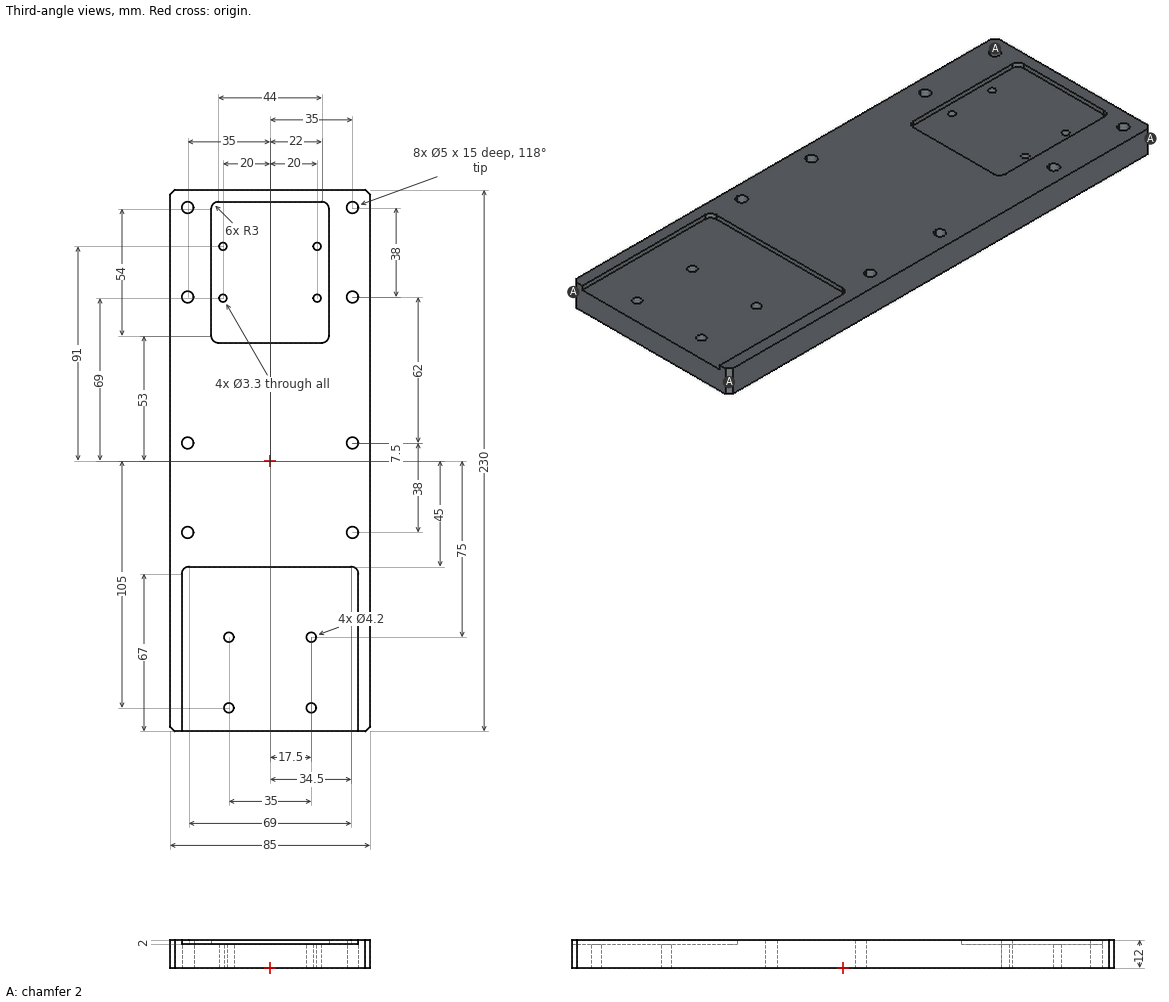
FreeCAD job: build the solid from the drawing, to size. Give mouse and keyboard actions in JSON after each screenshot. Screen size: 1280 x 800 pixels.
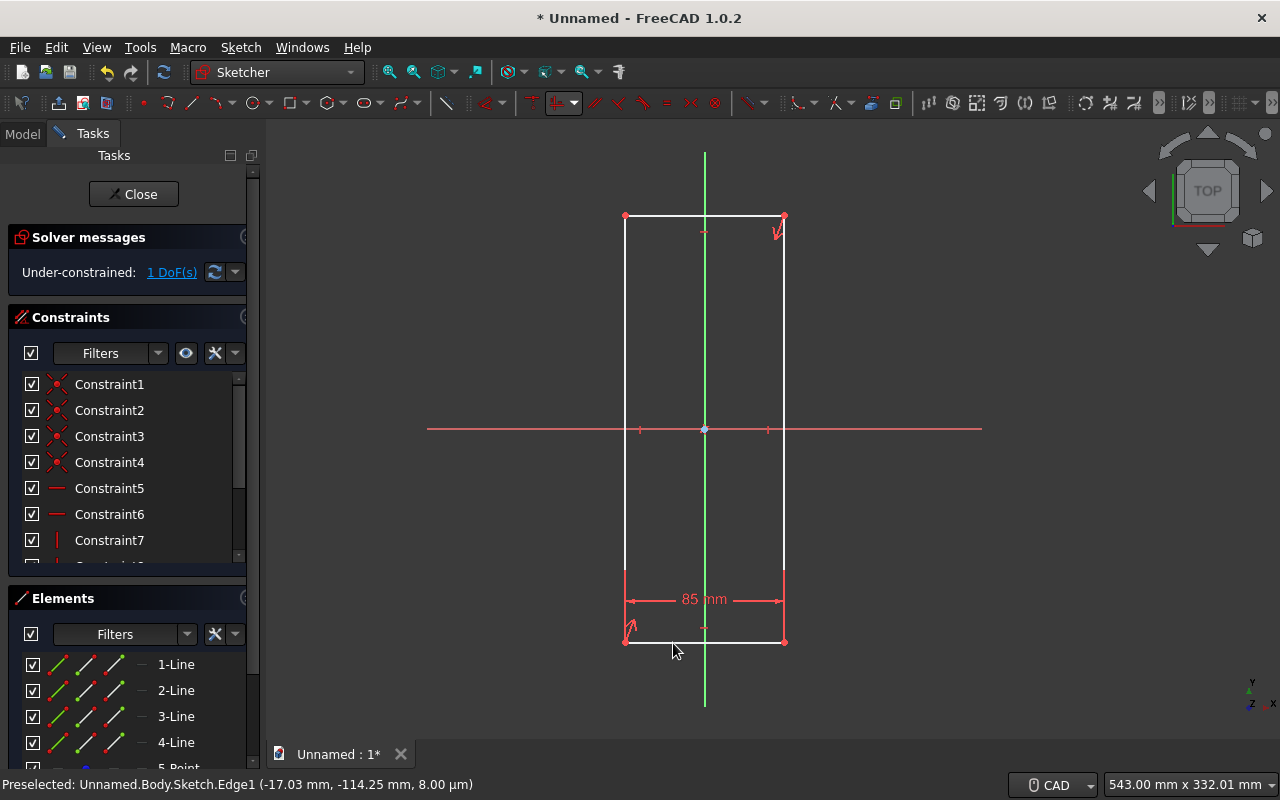
{"action": "left_click", "coordinate": [784, 515]}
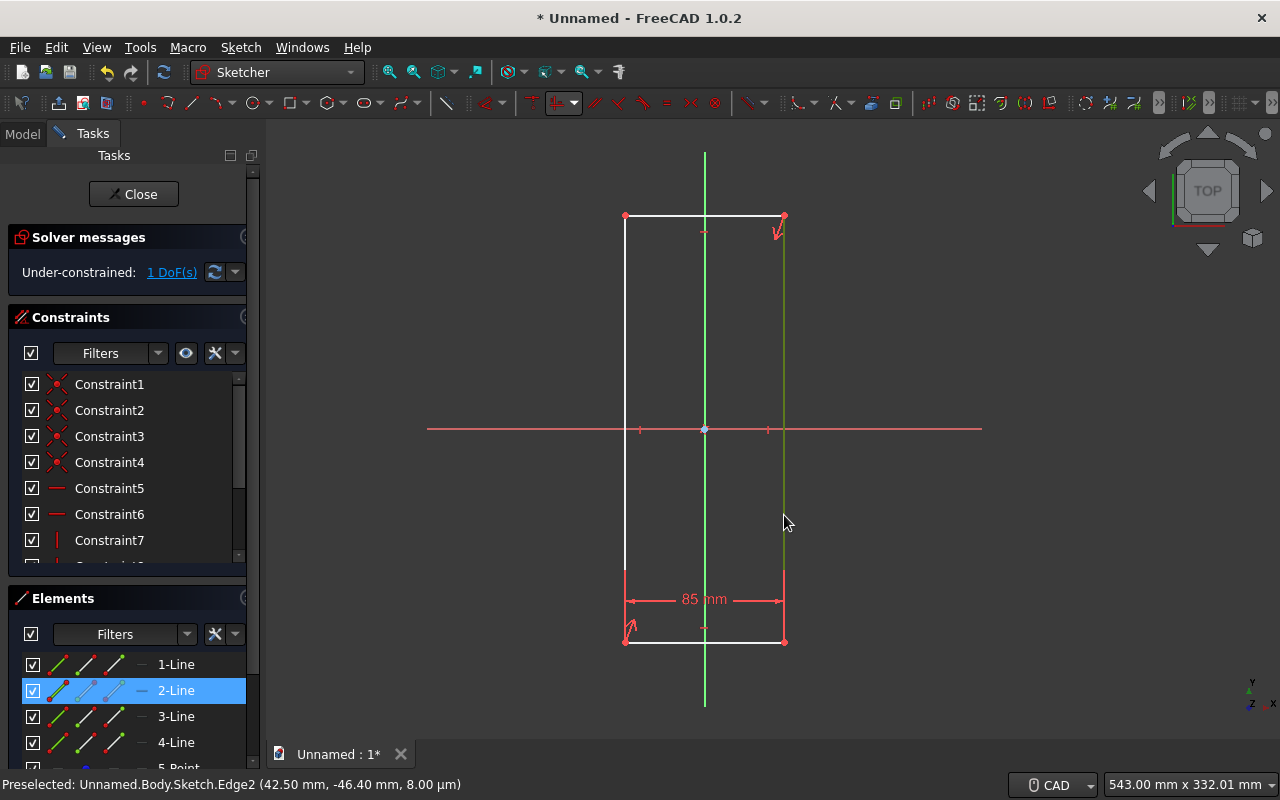
{"action": "key", "text": "i"}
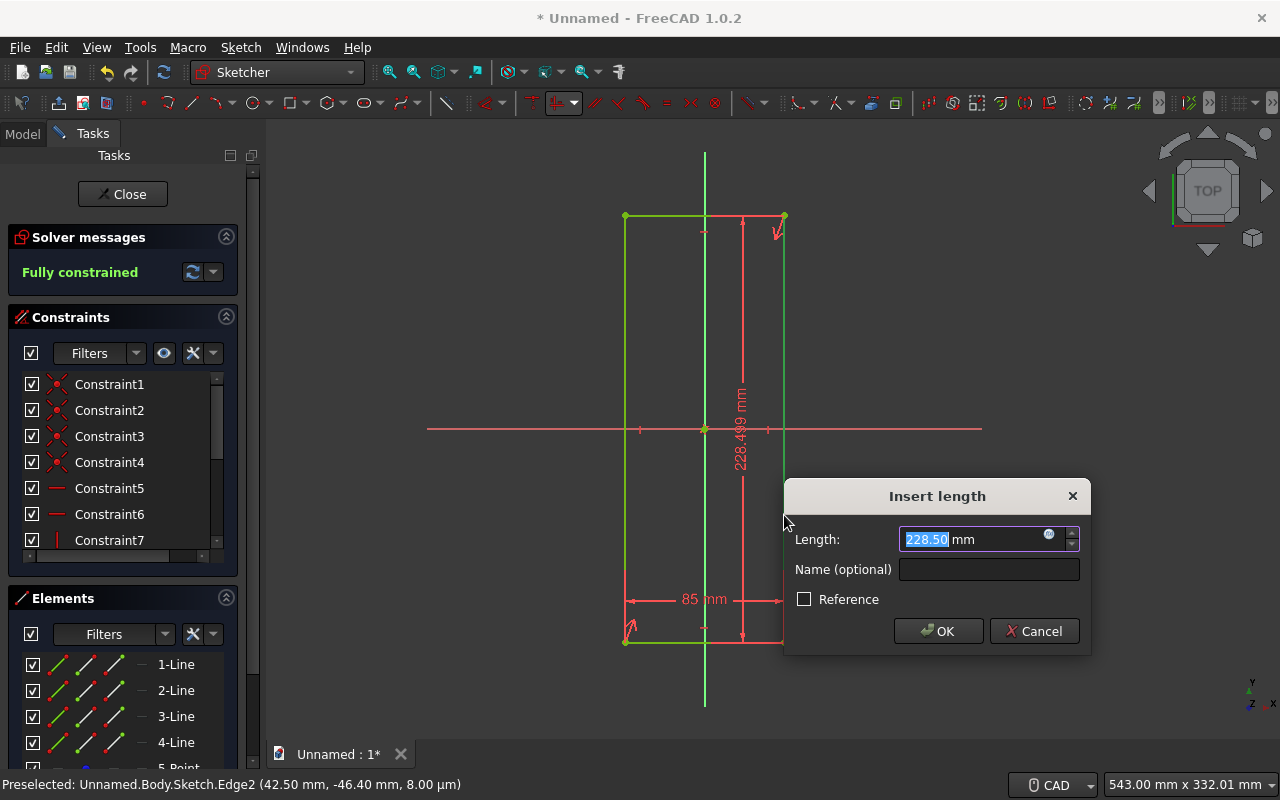
{"action": "type", "text": "230"}
{"action": "key", "text": "Return"}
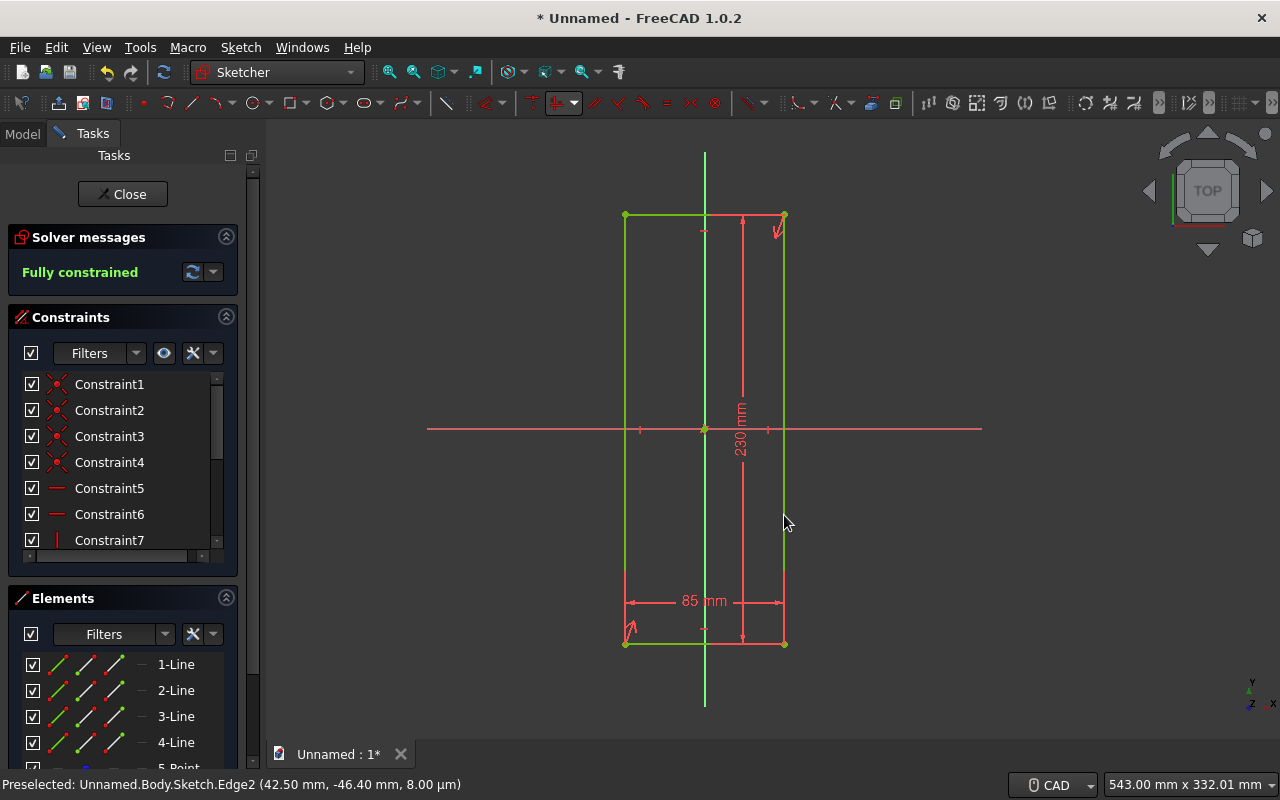
{"action": "left_click", "coordinate": [123, 194]}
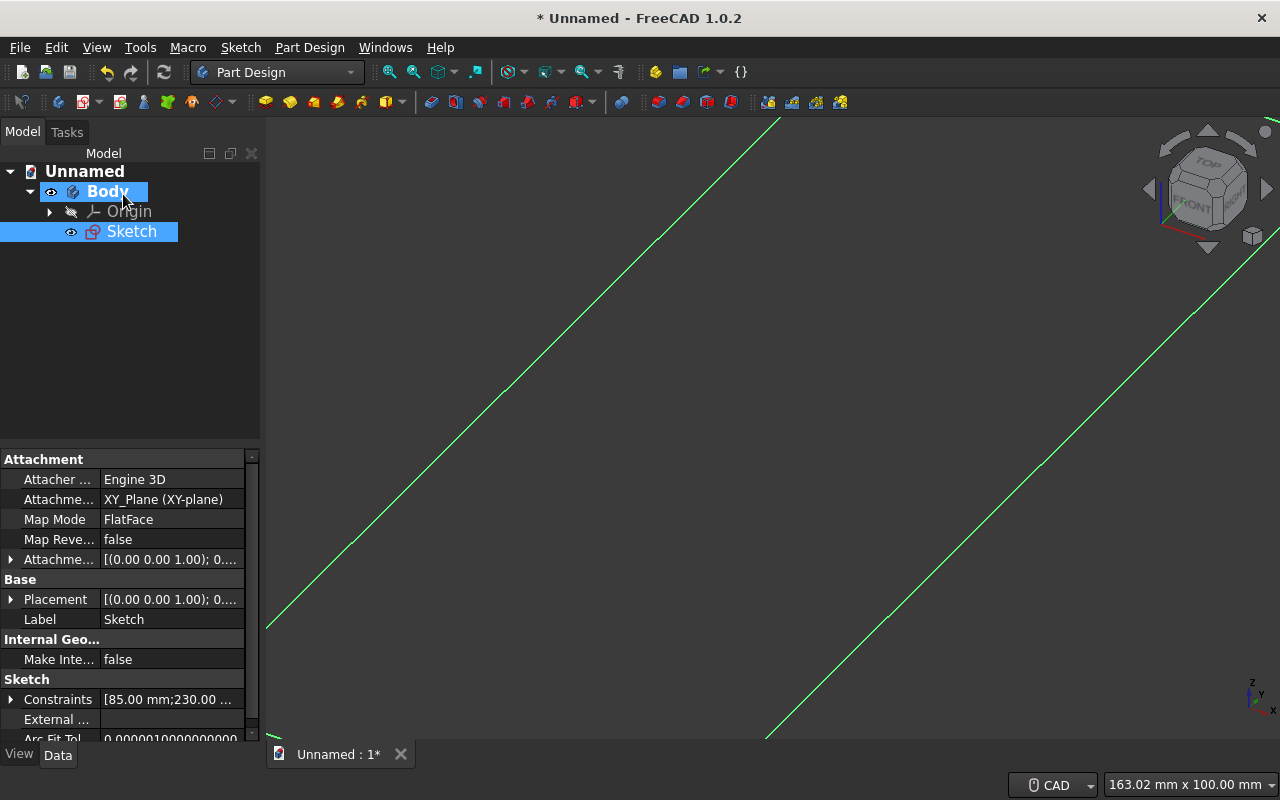
{"action": "left_click", "coordinate": [266, 102]}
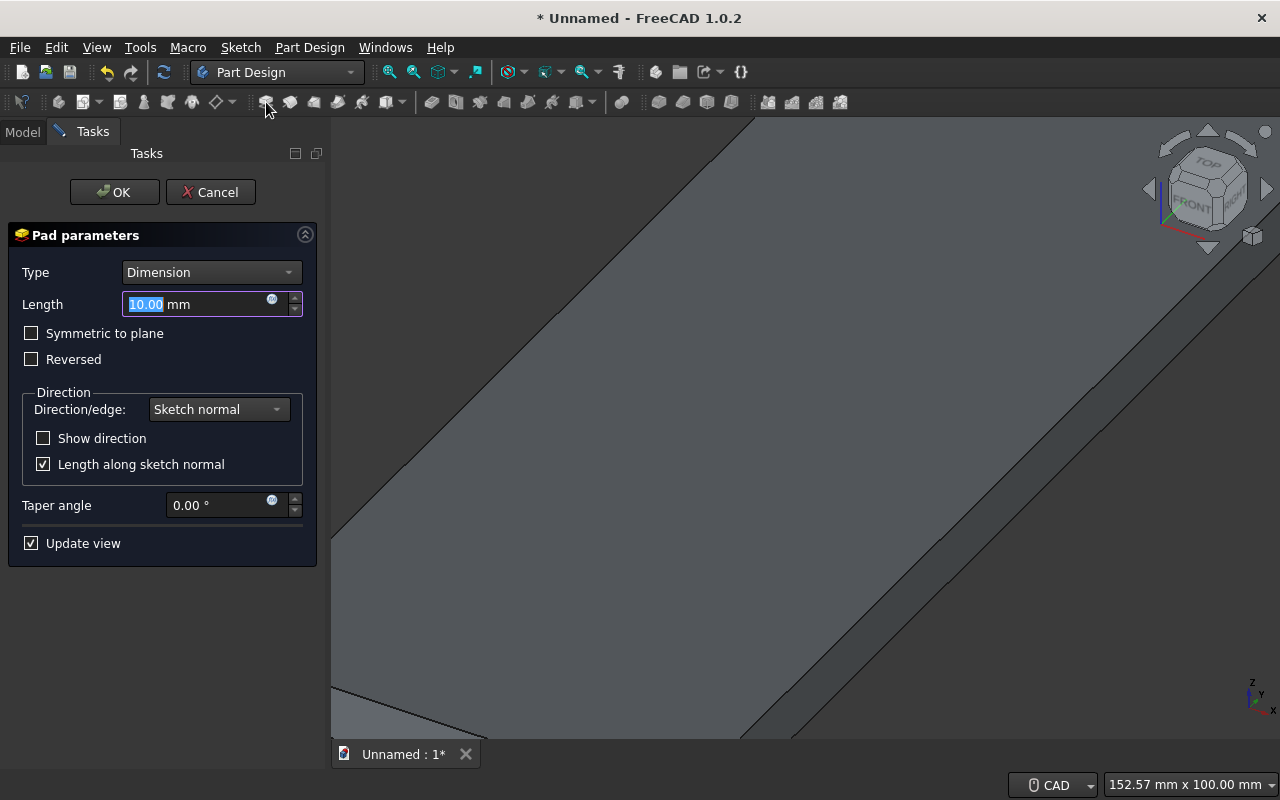
{"action": "type", "text": "12"}
{"action": "key", "text": "Tab"}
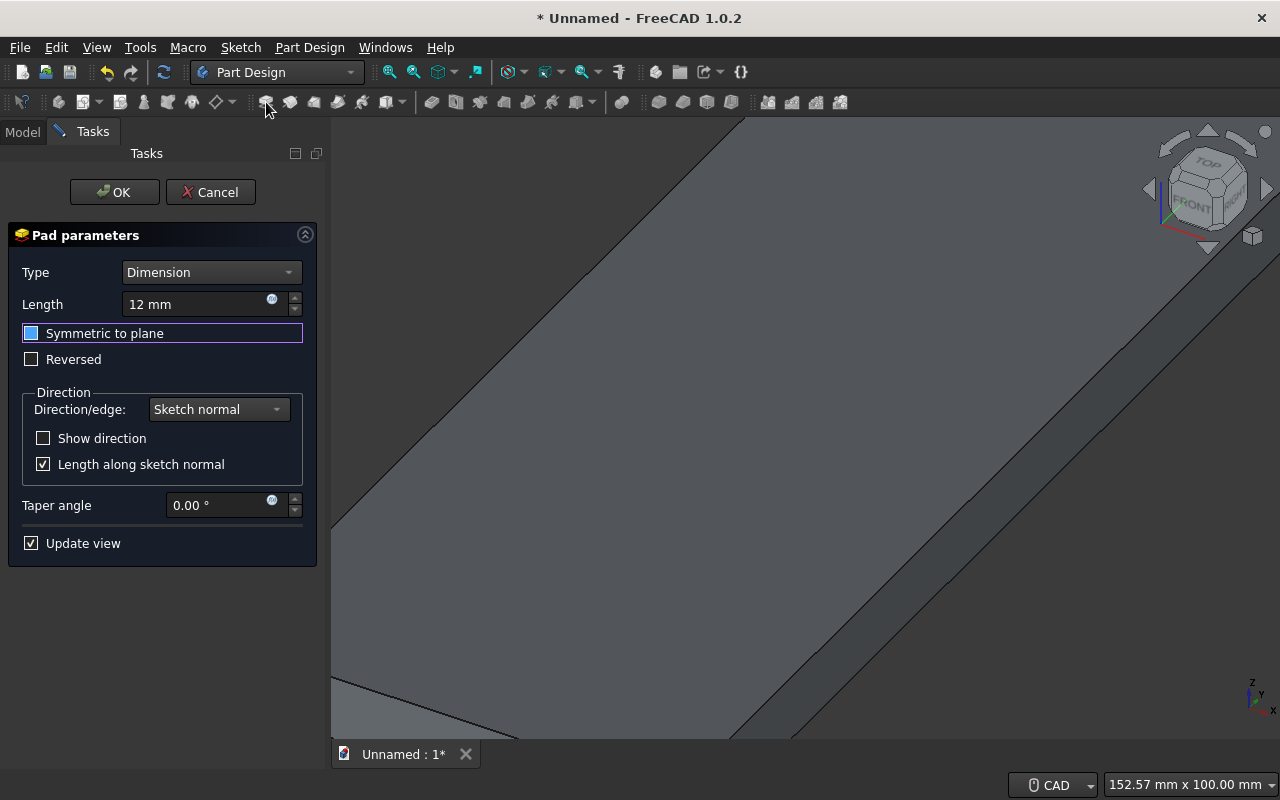
{"action": "left_click", "coordinate": [115, 192]}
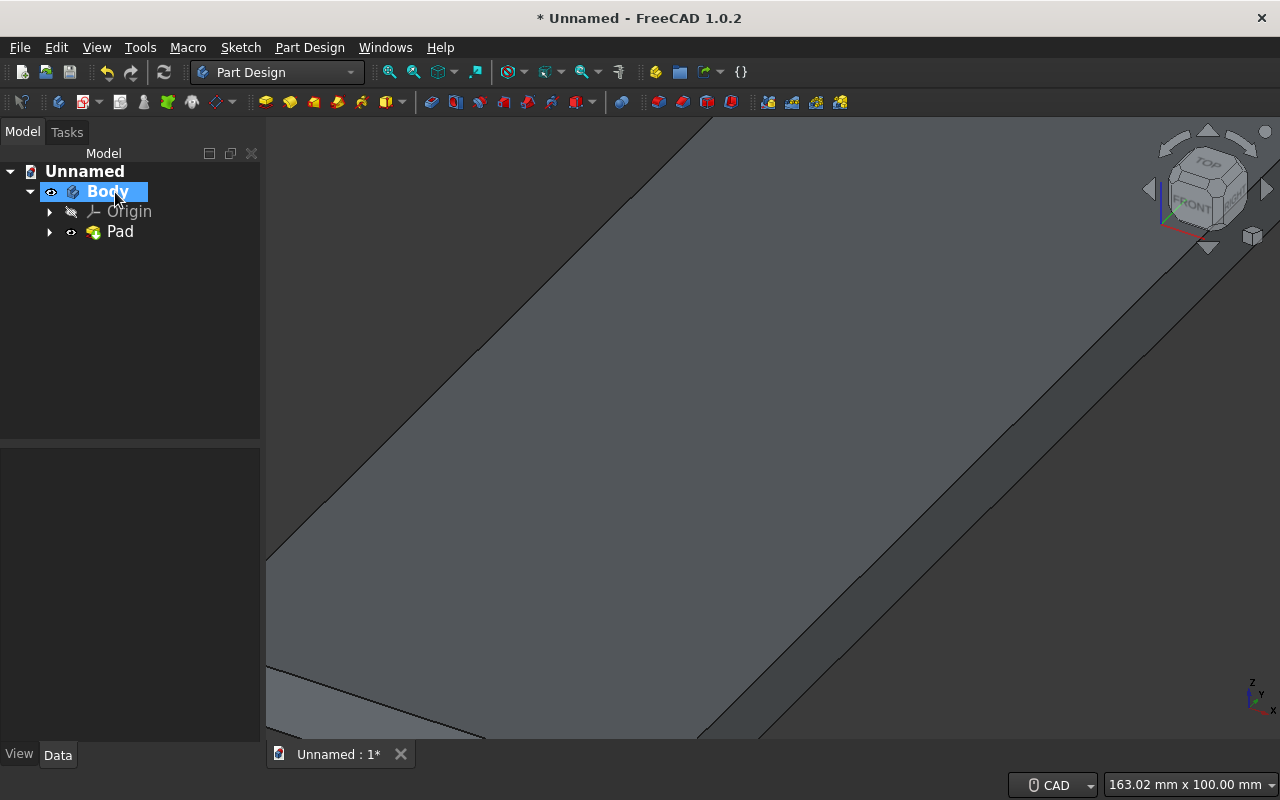
{"action": "key", "text": "v f"}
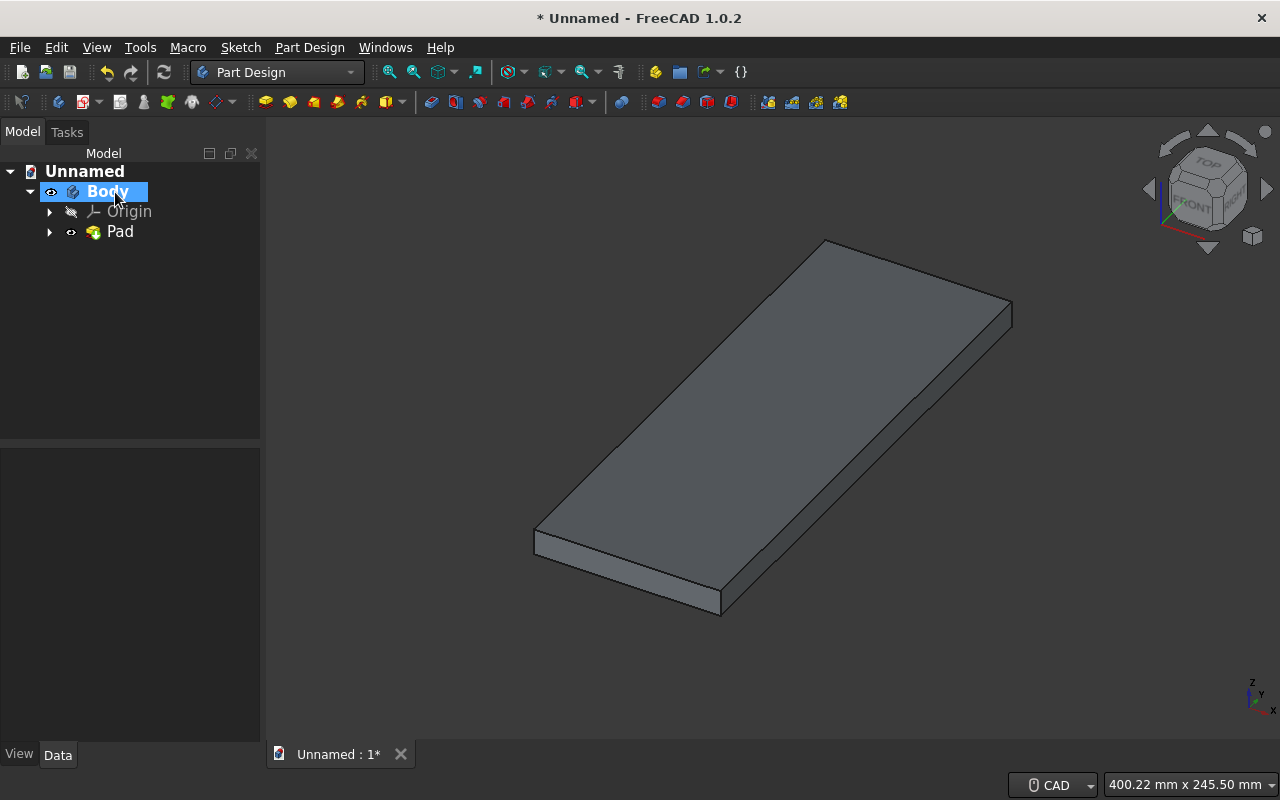
{"action": "left_click", "coordinate": [856, 332]}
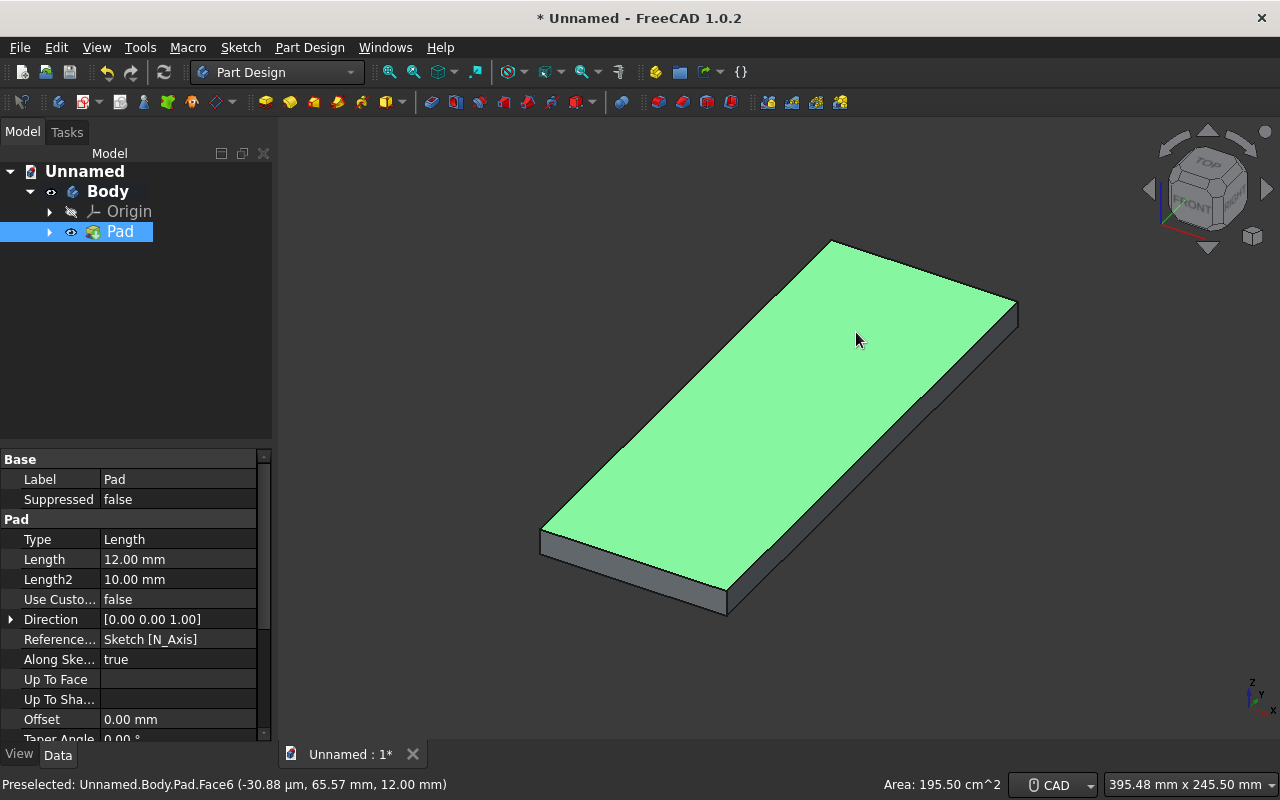
{"action": "left_click", "coordinate": [84, 102]}